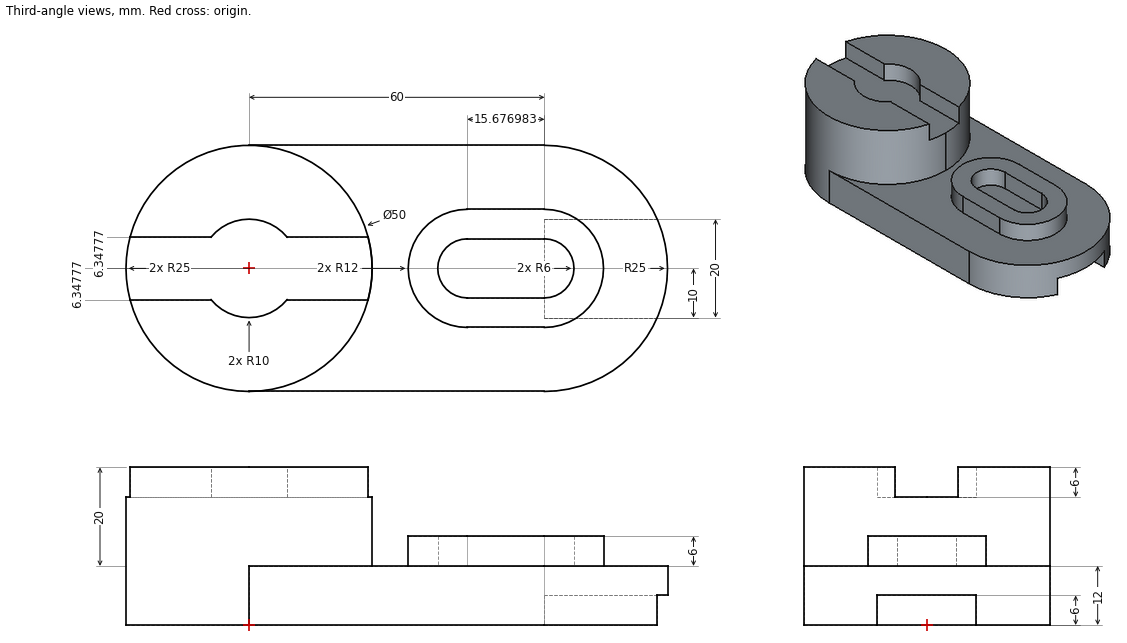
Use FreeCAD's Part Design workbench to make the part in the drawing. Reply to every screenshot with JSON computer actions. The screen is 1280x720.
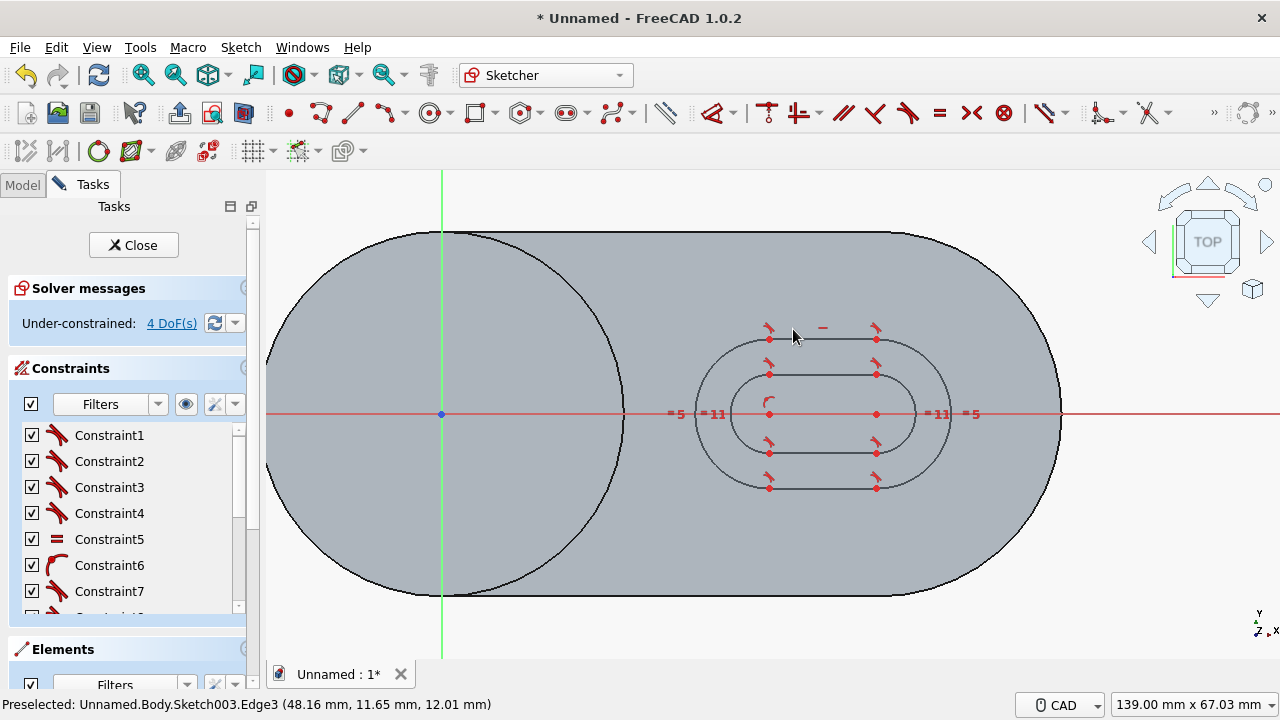
{"action": "key", "text": "d"}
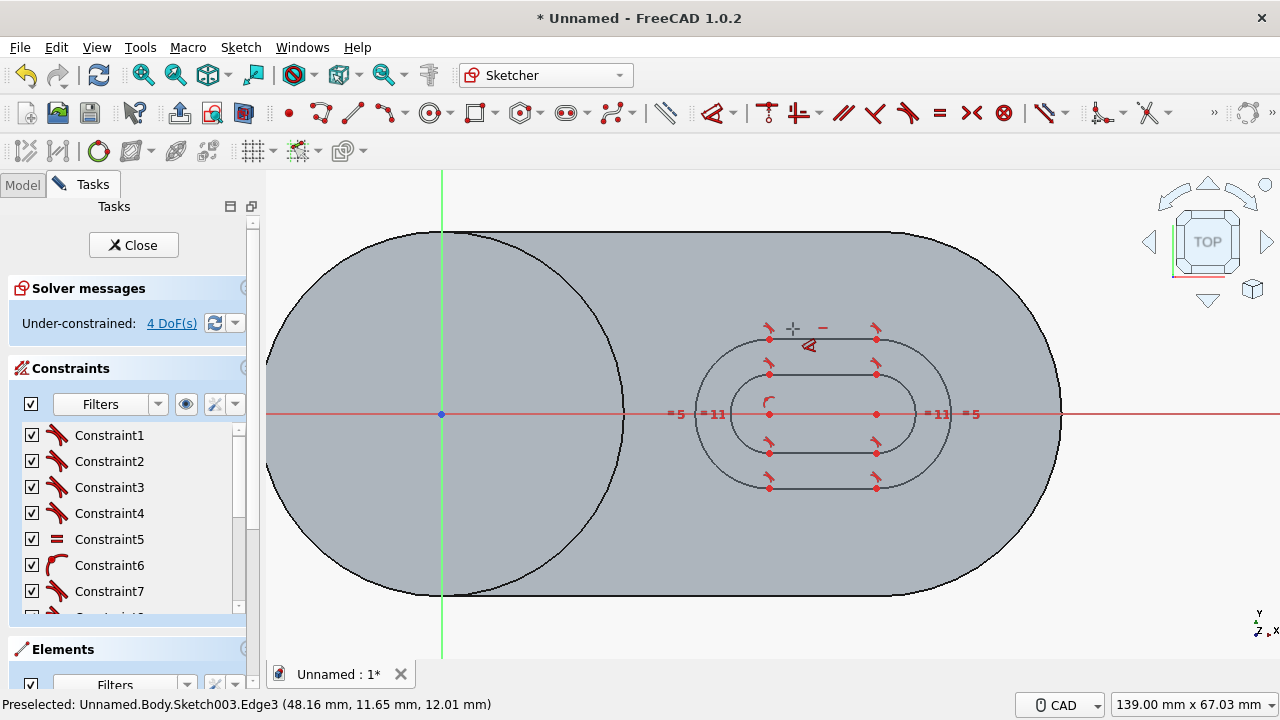
{"action": "left_click", "coordinate": [710, 370]}
{"action": "left_click", "coordinate": [684, 351]}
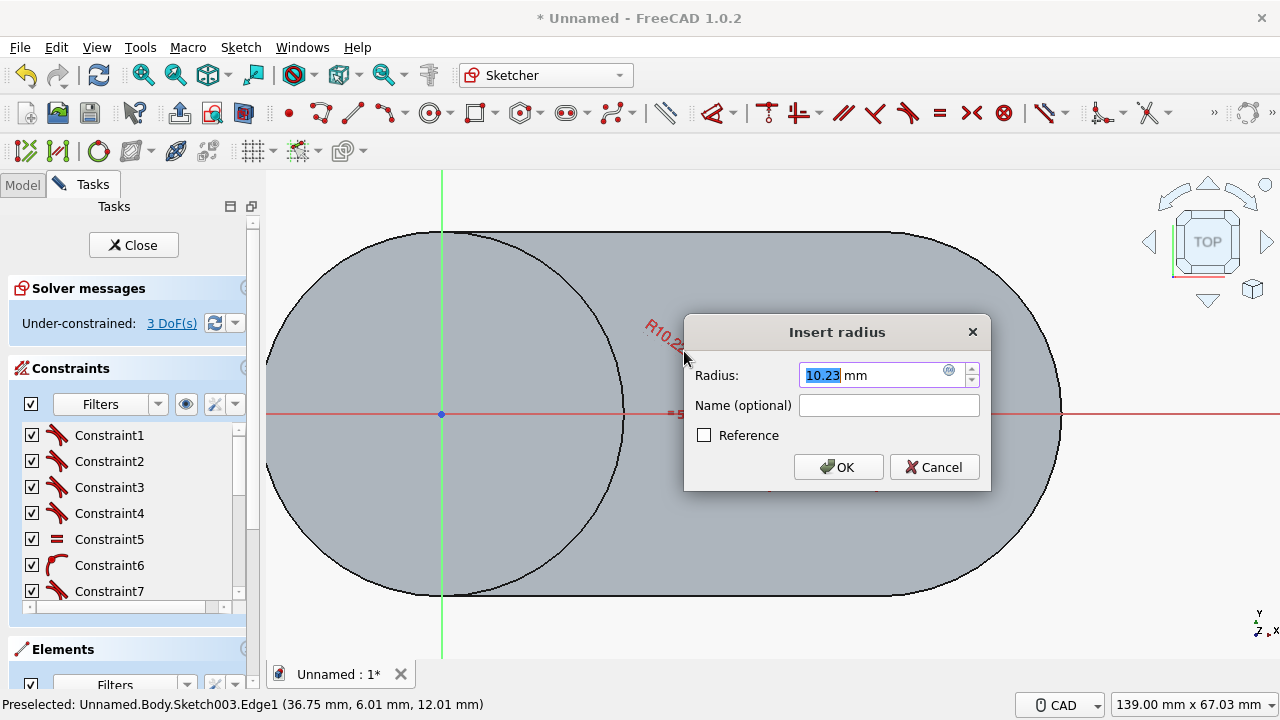
{"action": "type", "text": "12"}
{"action": "key", "text": "Return"}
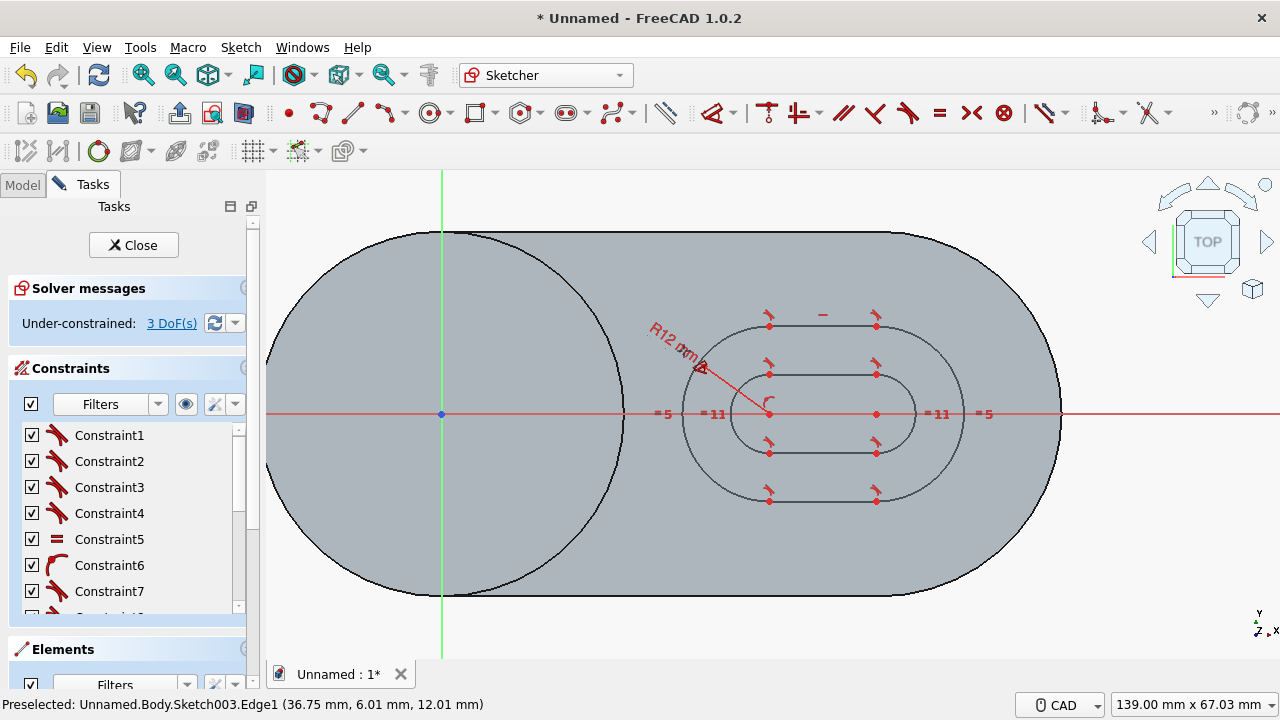
{"action": "left_click", "coordinate": [738, 391]}
{"action": "left_click", "coordinate": [712, 372]}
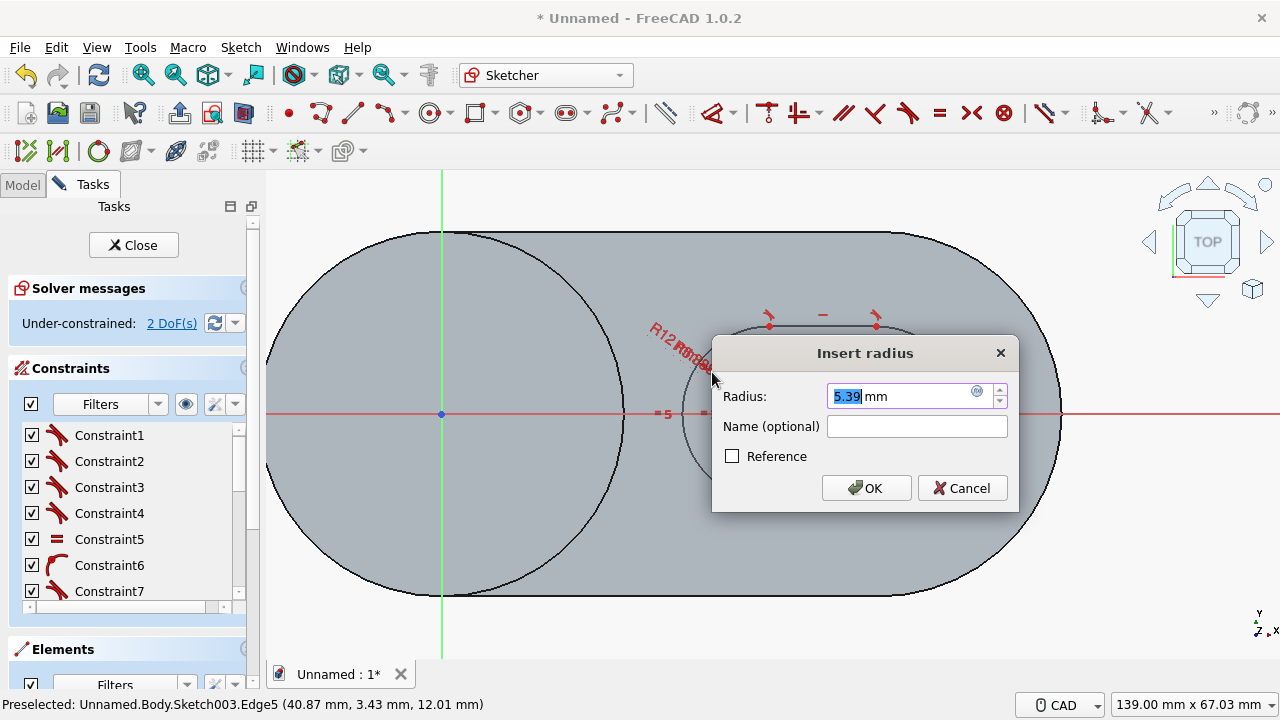
{"action": "type", "text": "6"}
{"action": "key", "text": "Return"}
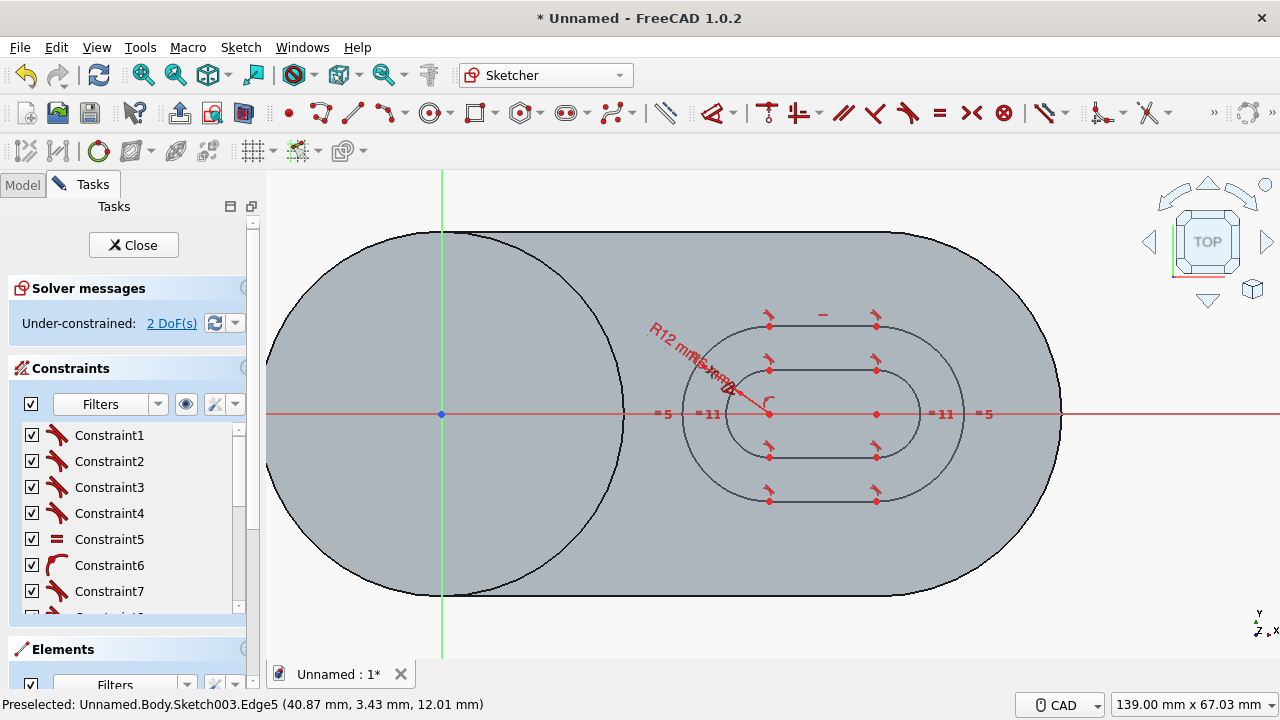
{"action": "left_click", "coordinate": [876, 502]}
{"action": "left_click", "coordinate": [659, 536]}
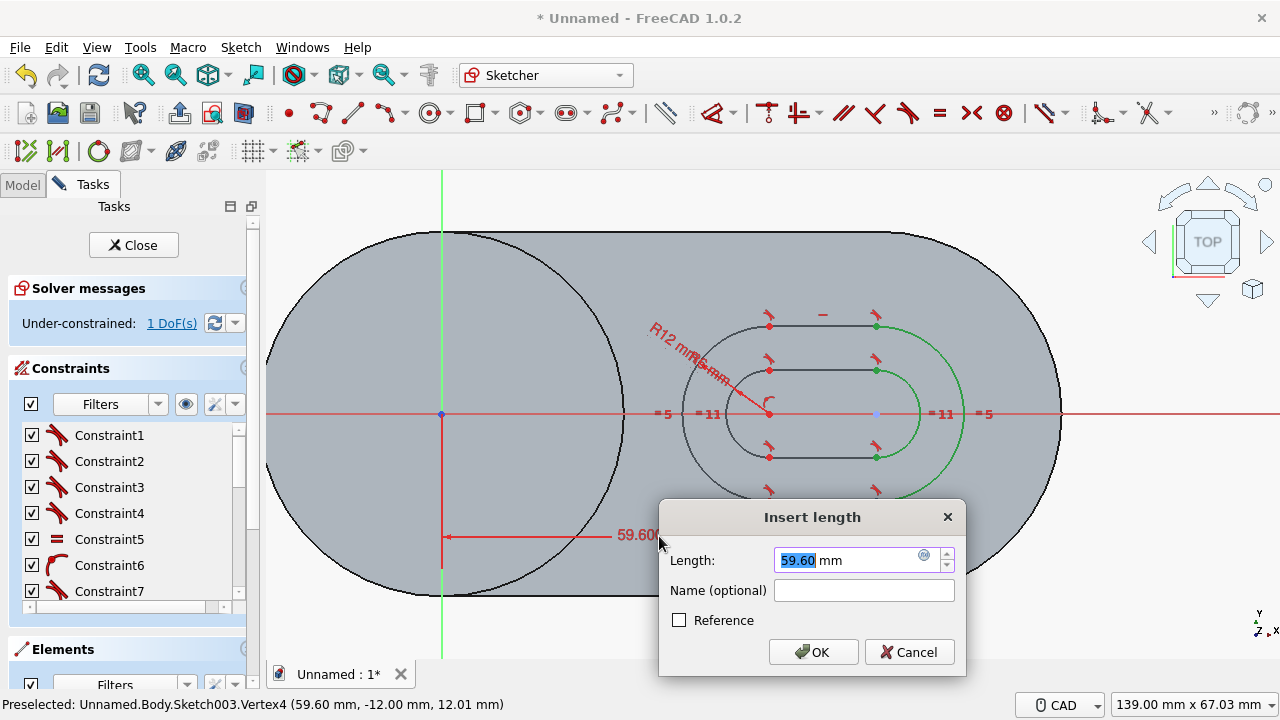
{"action": "type", "text": "60"}
{"action": "key", "text": "Return"}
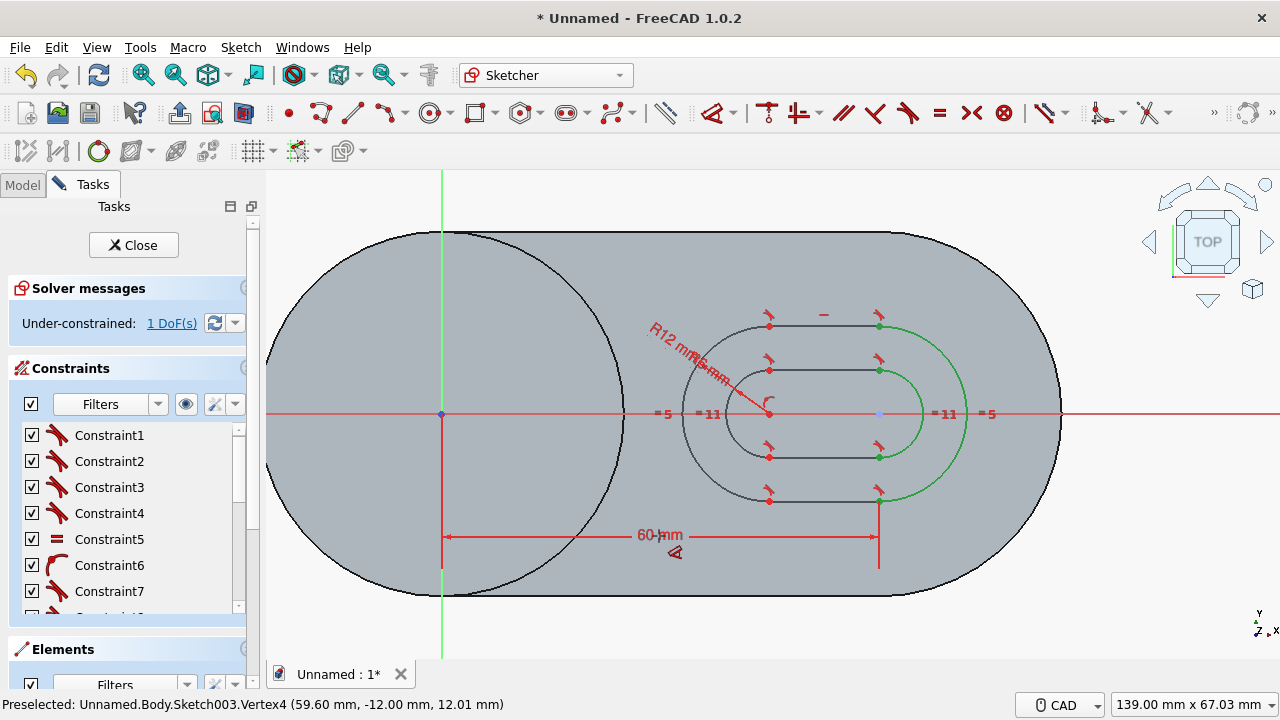
{"action": "left_click", "coordinate": [803, 326]}
{"action": "left_click", "coordinate": [825, 292]}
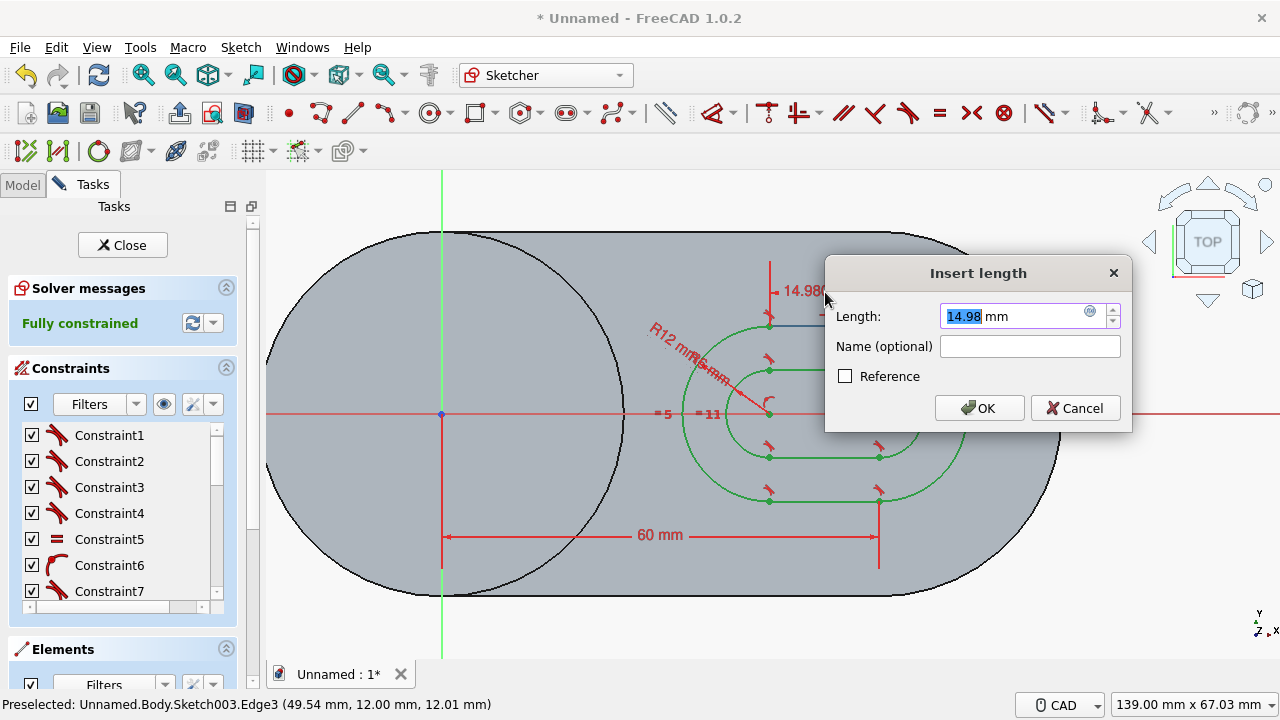
{"action": "type", "text": "15.676983"}
{"action": "key", "text": "Return"}
{"action": "key", "text": "Escape"}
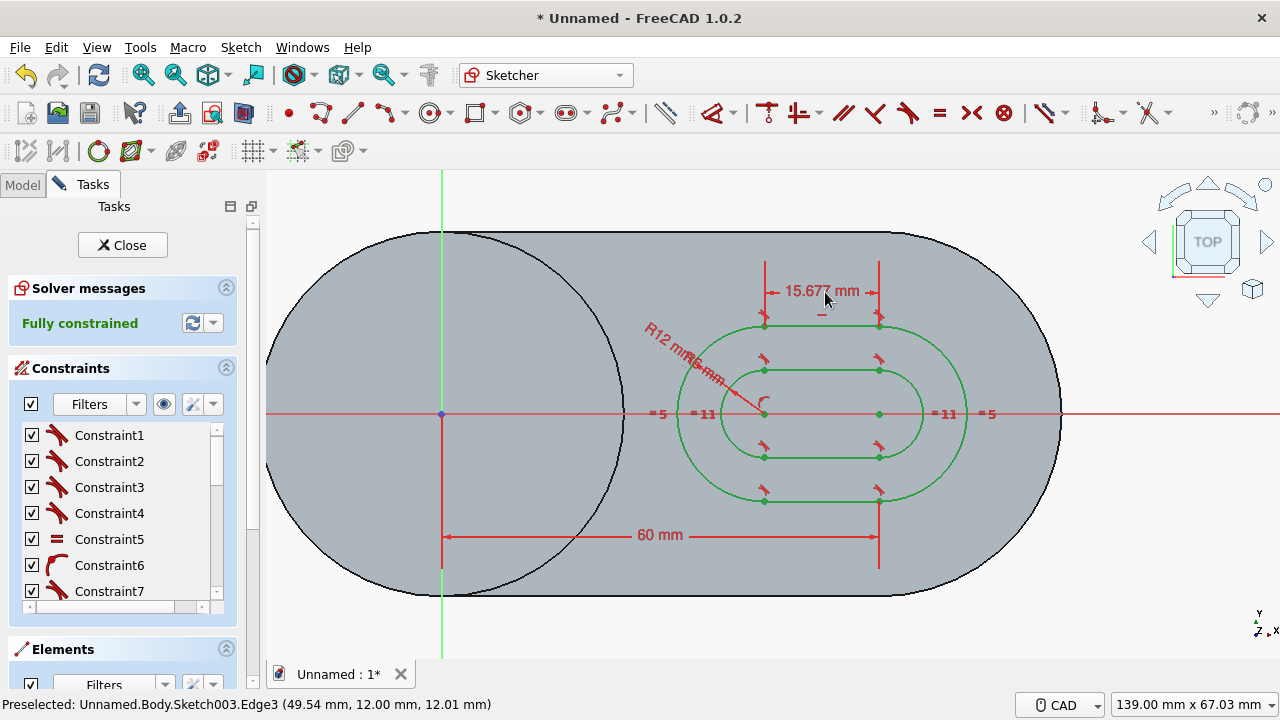
{"action": "left_click", "coordinate": [123, 245]}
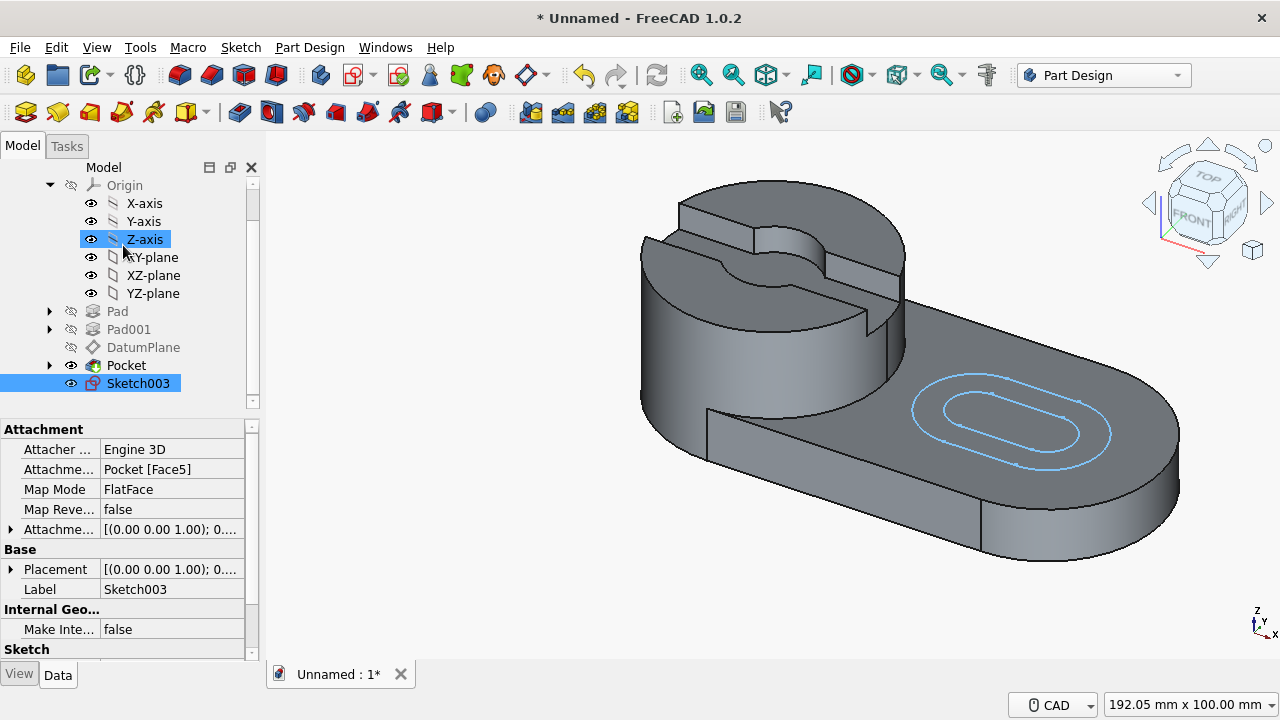
{"action": "left_click", "coordinate": [26, 112]}